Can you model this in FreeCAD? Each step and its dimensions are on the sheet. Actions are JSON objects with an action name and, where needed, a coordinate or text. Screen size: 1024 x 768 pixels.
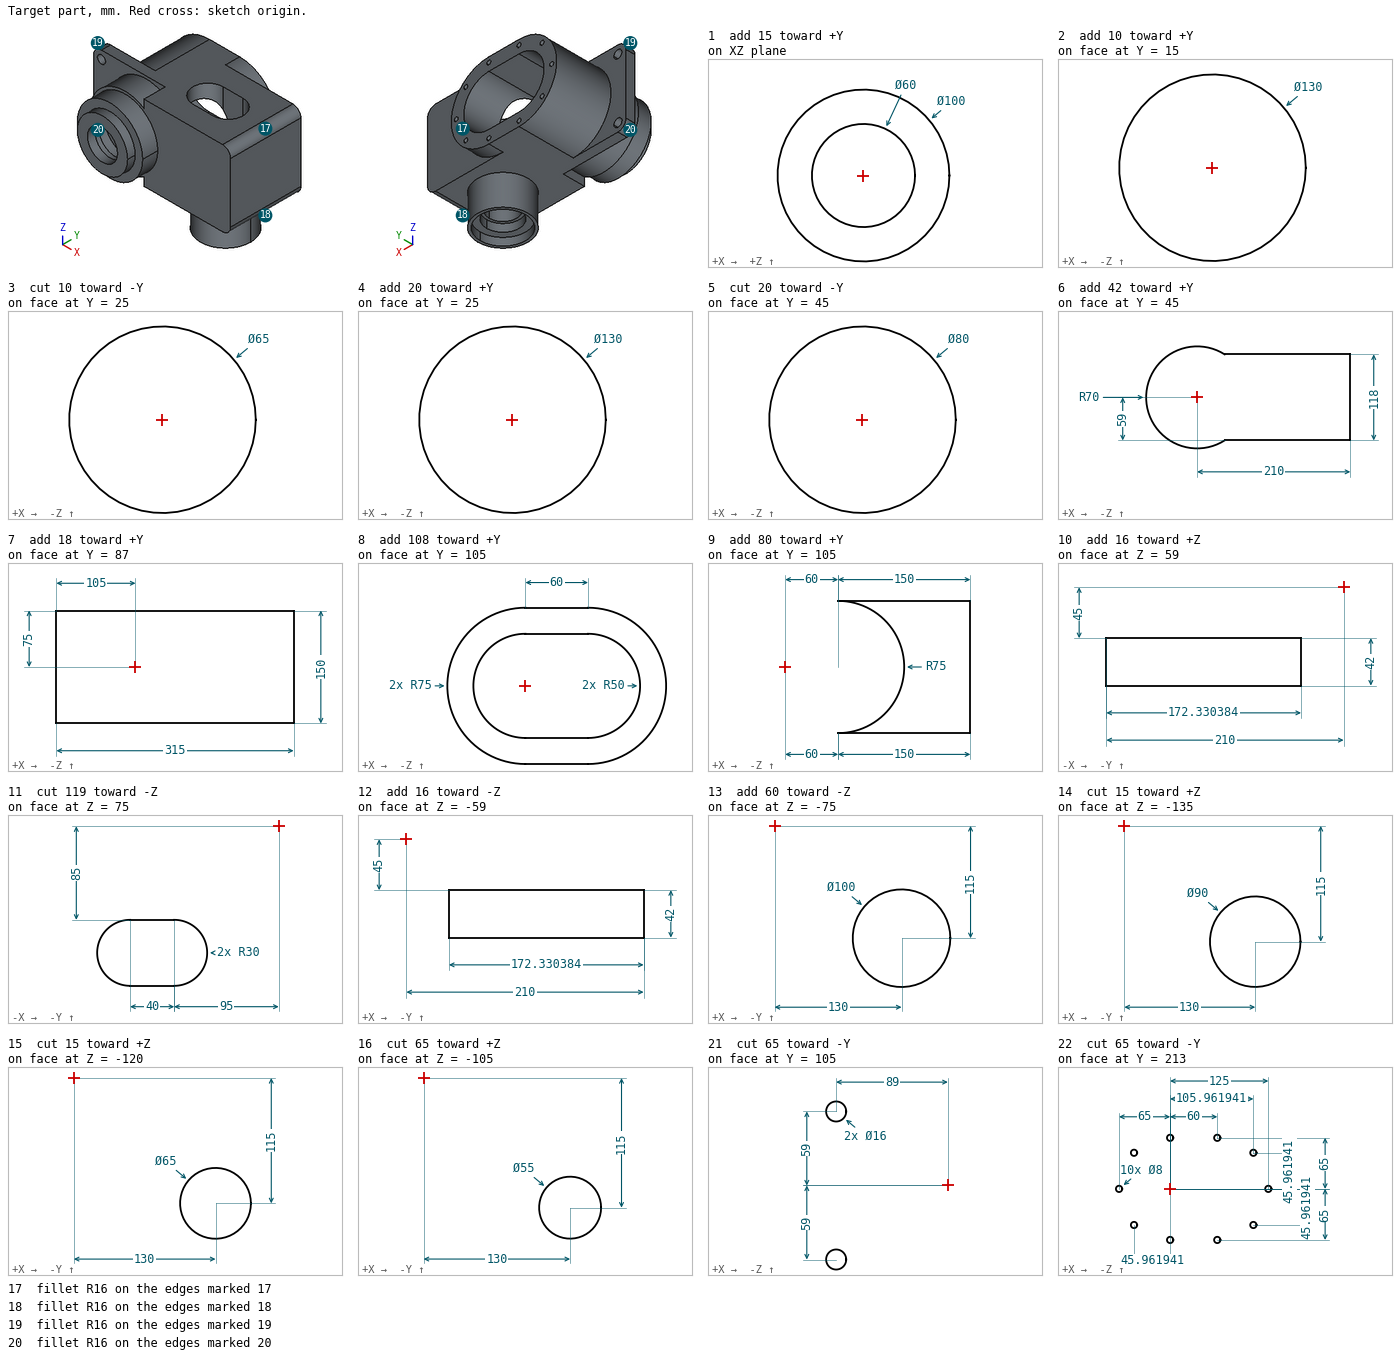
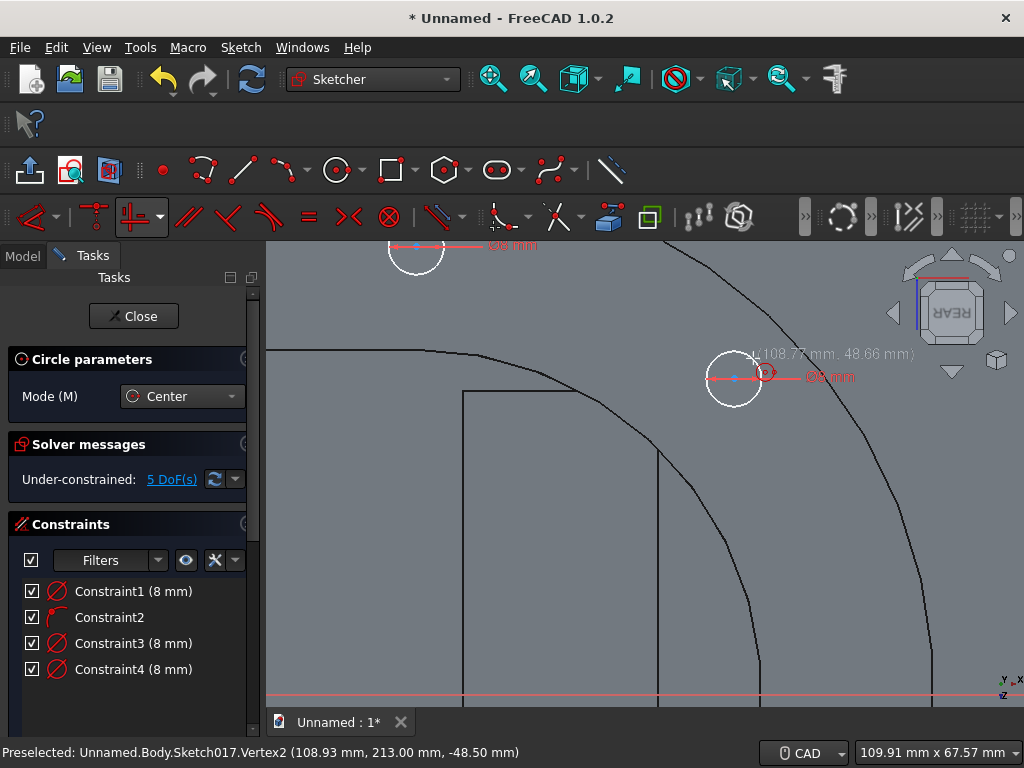
{"action": "scroll", "coordinate": [735, 379], "scroll_direction": "down", "scroll_amount": 6}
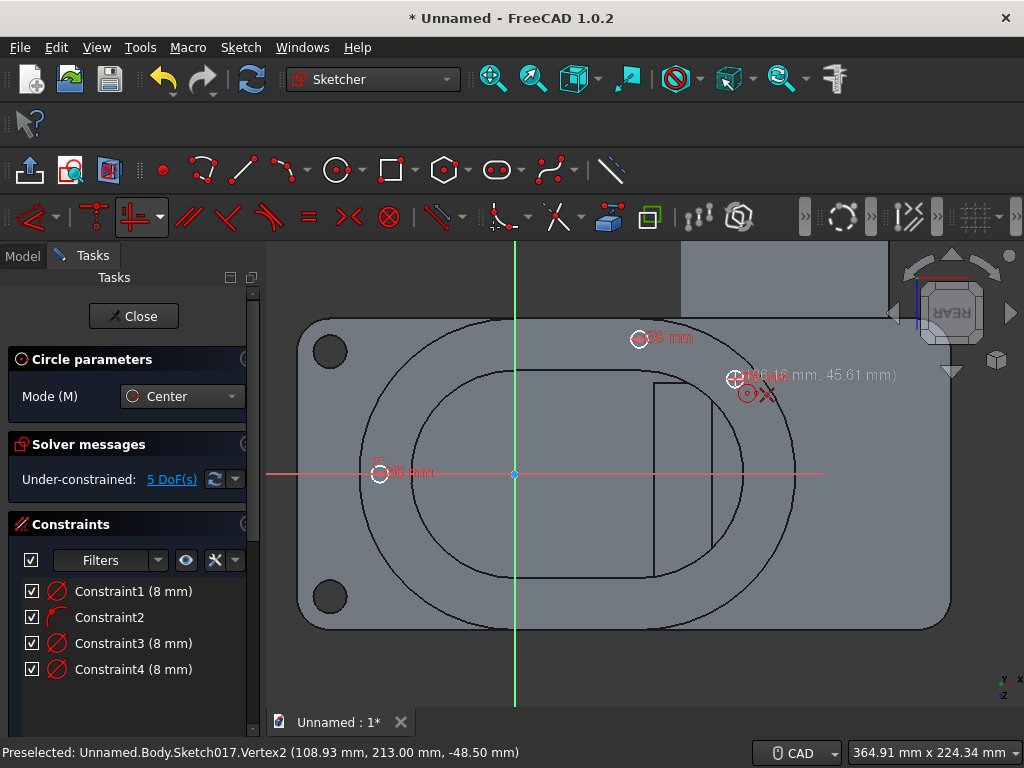
{"action": "scroll", "coordinate": [775, 474], "scroll_direction": "up", "scroll_amount": 6}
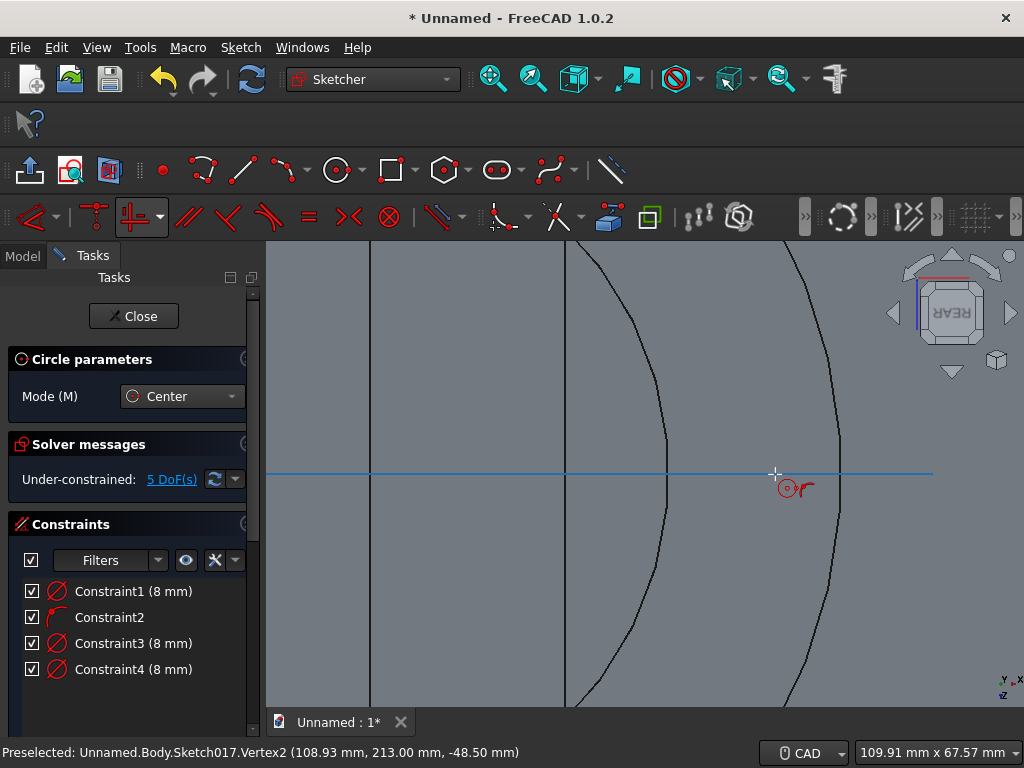
{"action": "left_click", "coordinate": [772, 474]}
{"action": "mouse_move", "coordinate": [792, 454]}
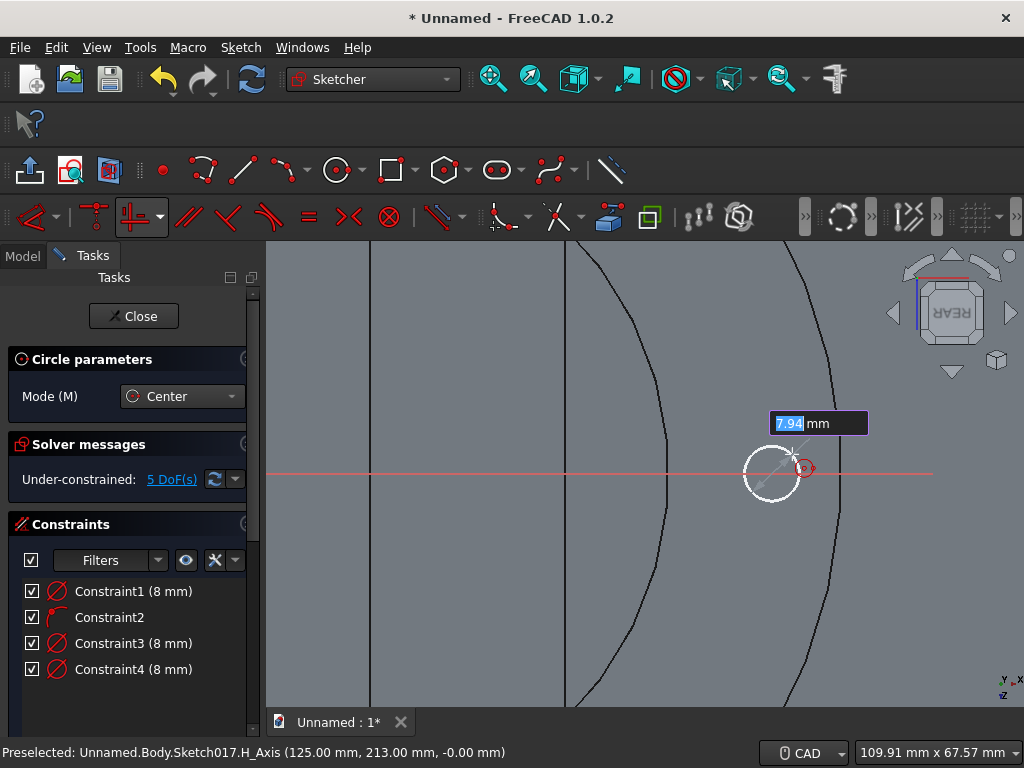
{"action": "type", "text": "8"}
{"action": "key", "text": "Return"}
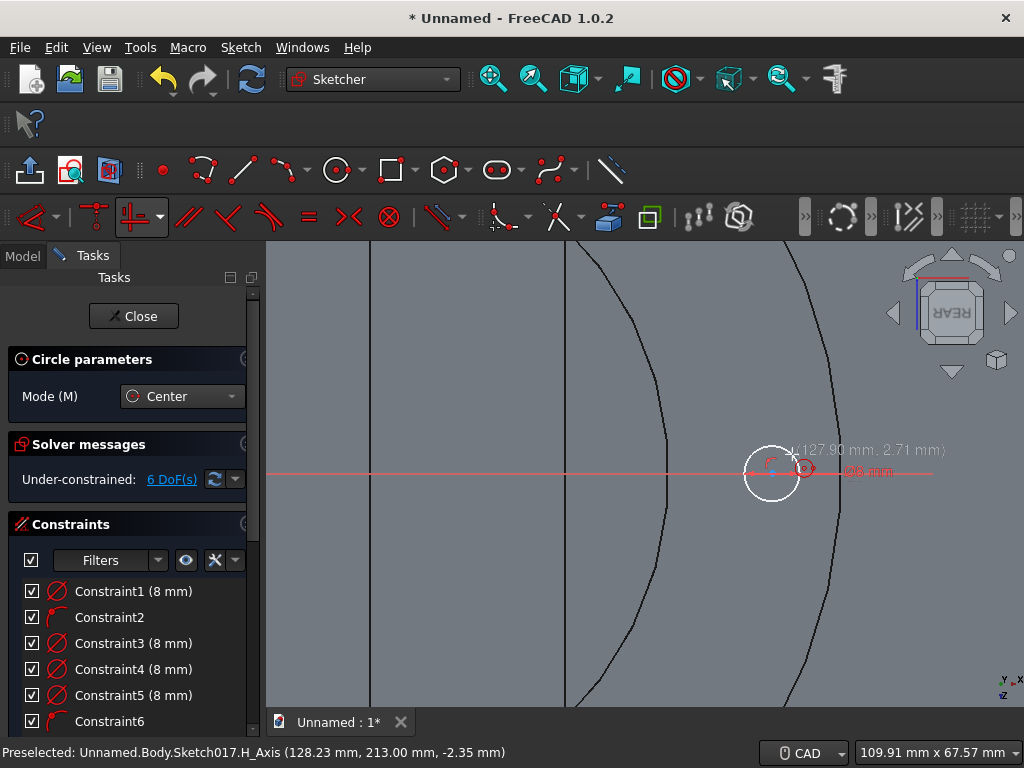
{"action": "scroll", "coordinate": [775, 474], "scroll_direction": "down", "scroll_amount": 6}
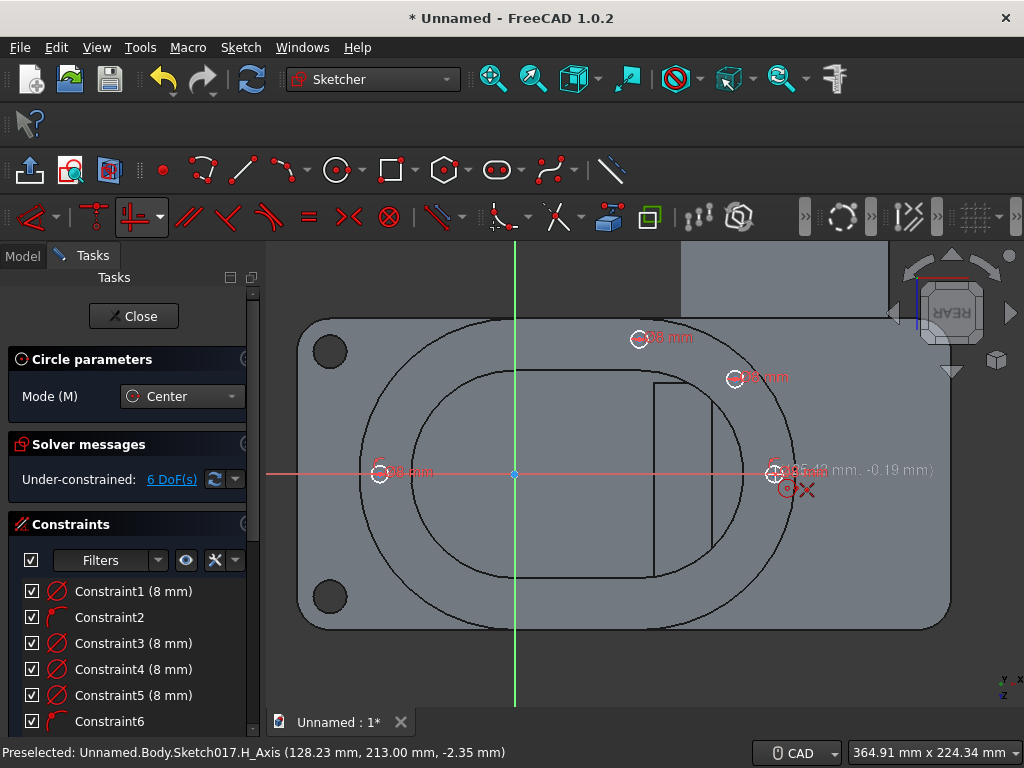
{"action": "scroll", "coordinate": [735, 570], "scroll_direction": "up", "scroll_amount": 6}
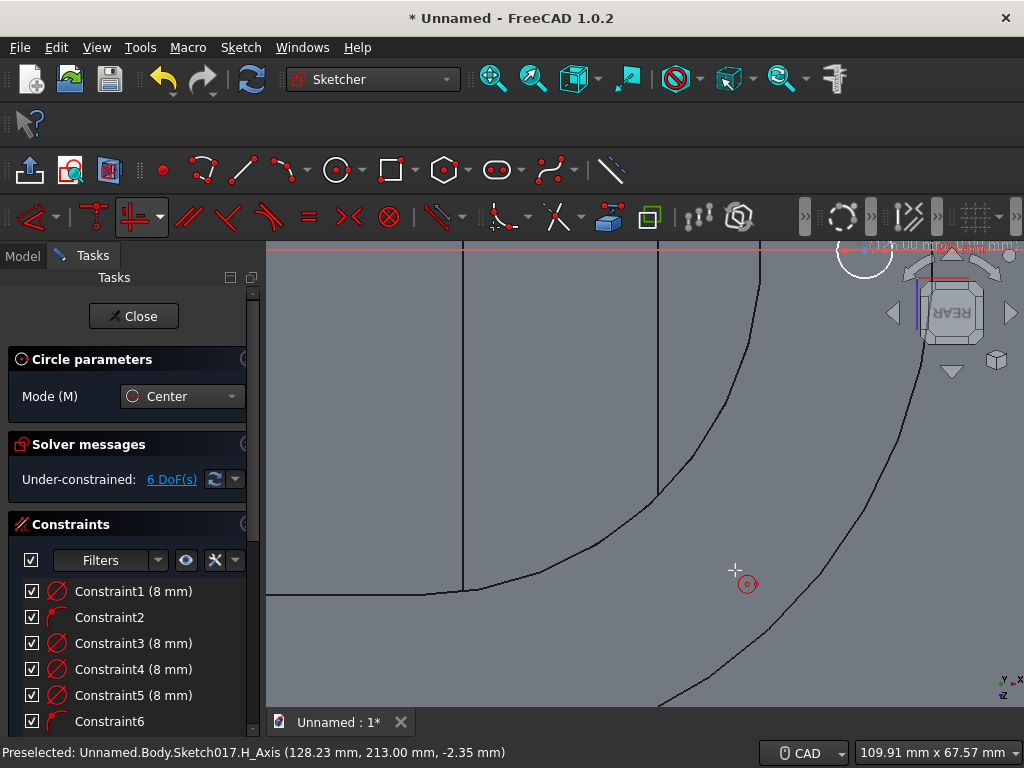
{"action": "left_click", "coordinate": [734, 567]}
{"action": "mouse_move", "coordinate": [753, 548]}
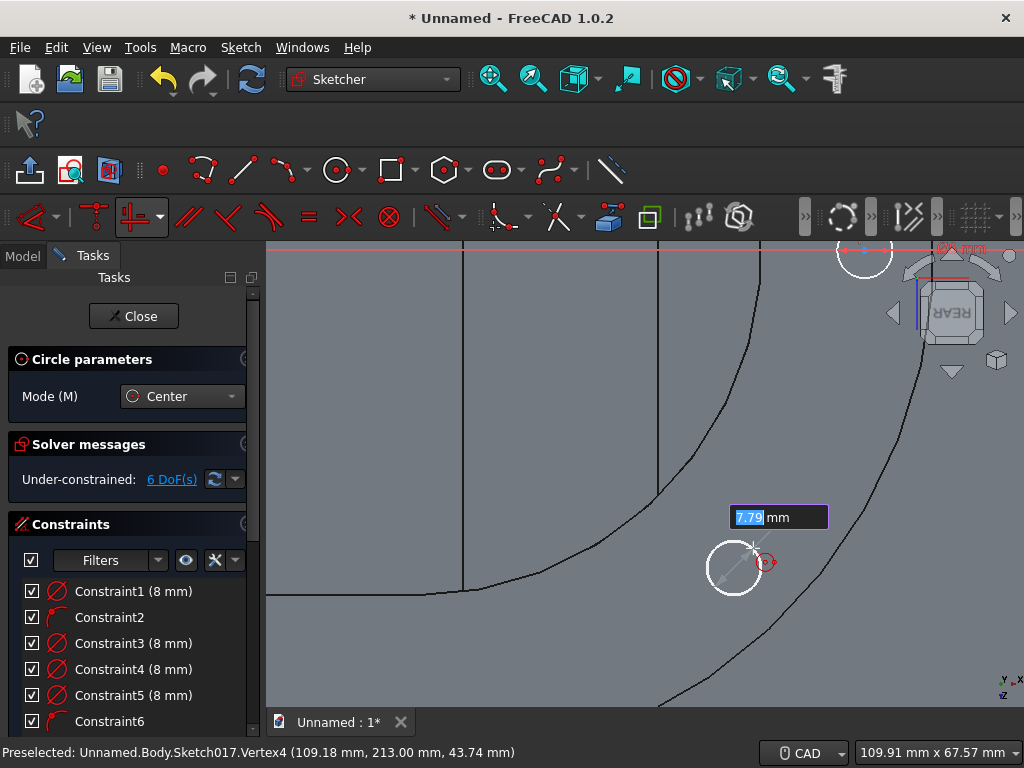
{"action": "type", "text": "8"}
{"action": "key", "text": "Return"}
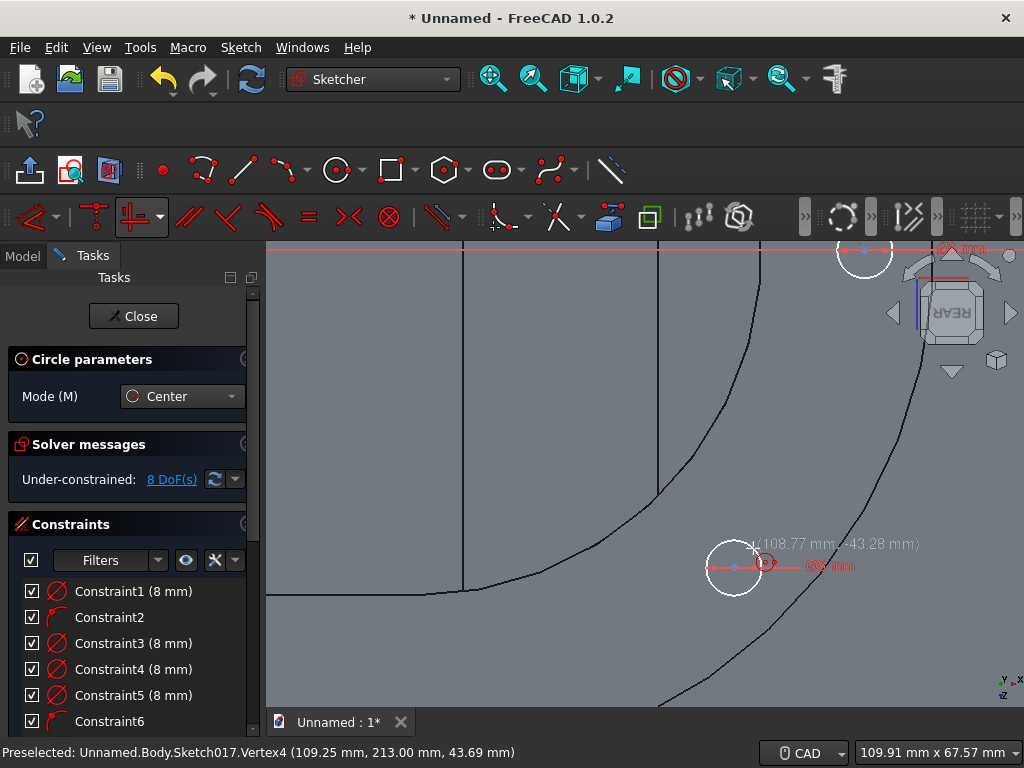
{"action": "scroll", "coordinate": [735, 570], "scroll_direction": "down", "scroll_amount": 6}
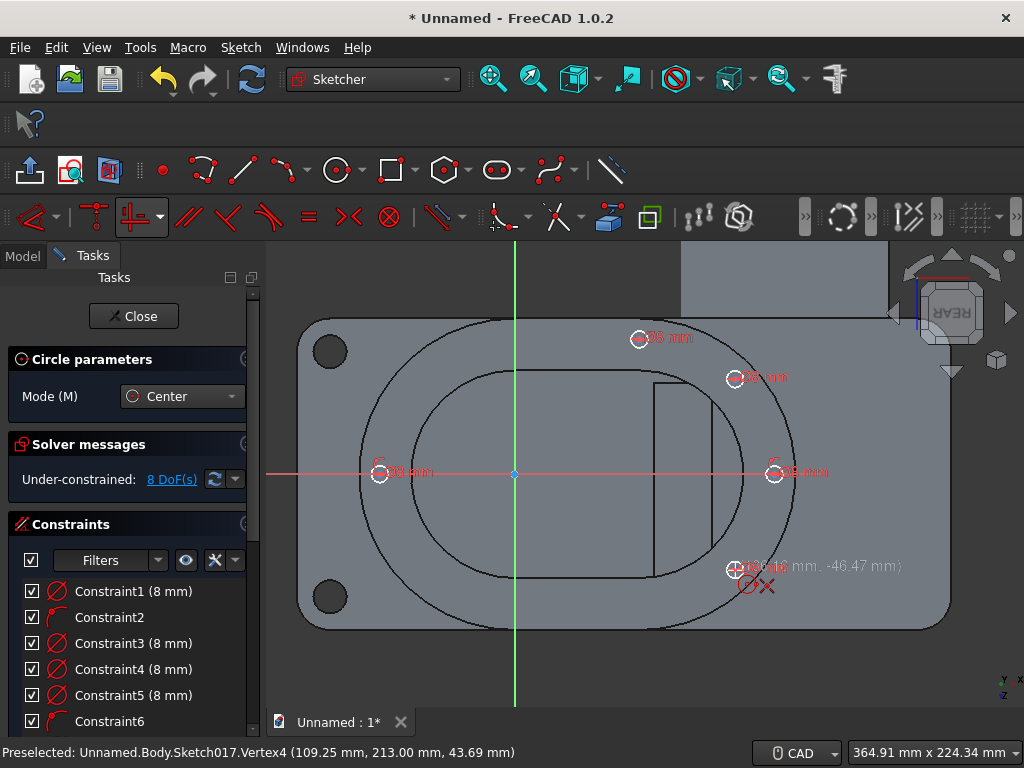
{"action": "scroll", "coordinate": [419, 570], "scroll_direction": "up", "scroll_amount": 6}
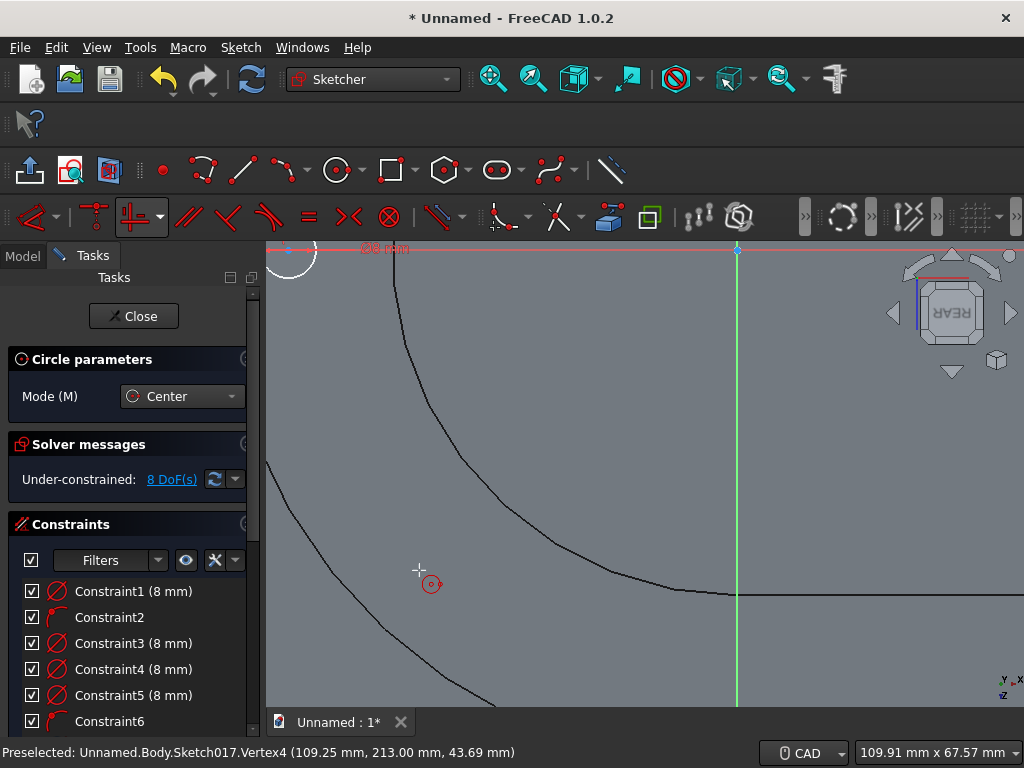
{"action": "left_click", "coordinate": [420, 567]}
{"action": "mouse_move", "coordinate": [440, 548]}